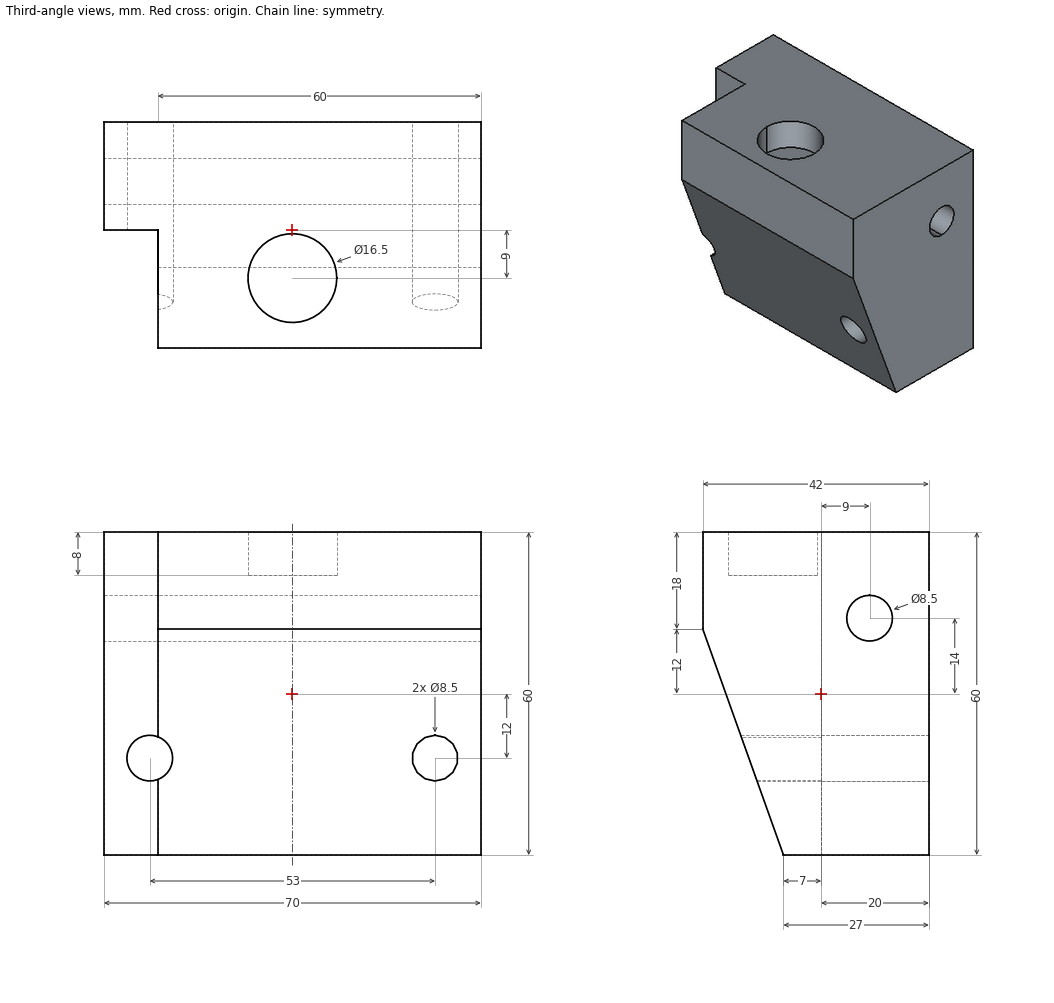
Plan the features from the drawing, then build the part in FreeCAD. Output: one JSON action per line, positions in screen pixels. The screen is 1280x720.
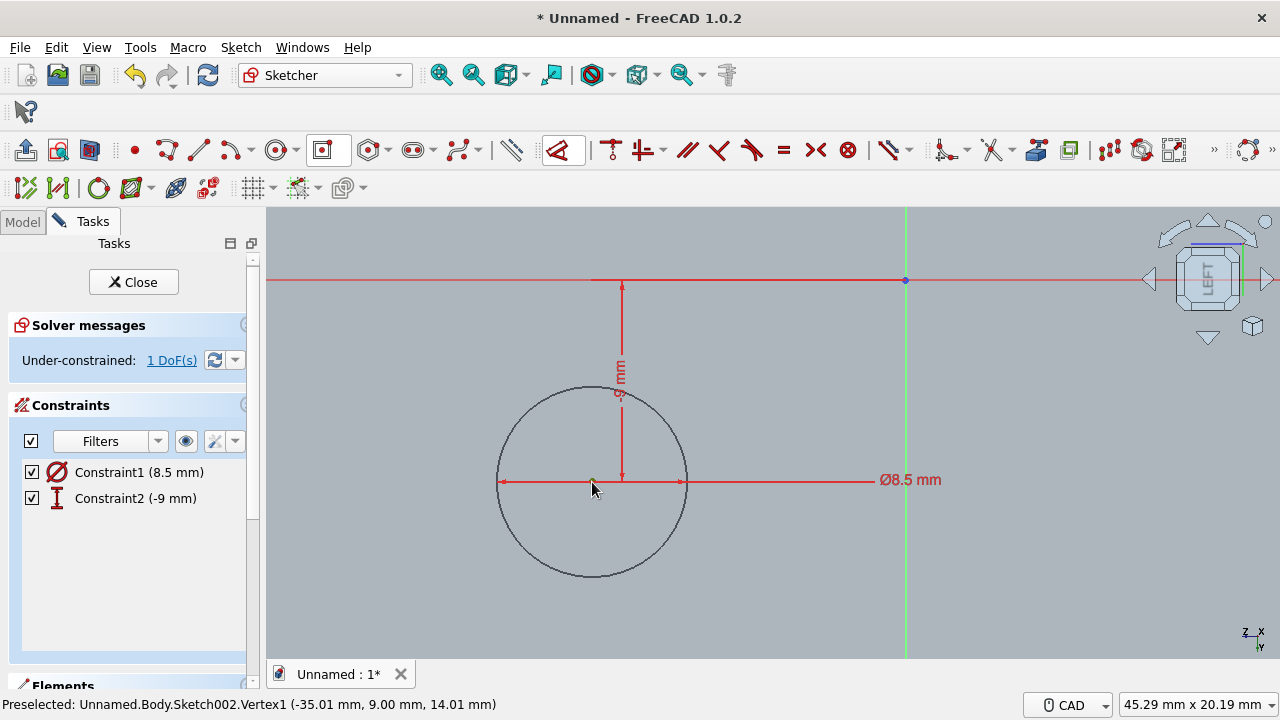
{"action": "key", "text": "l"}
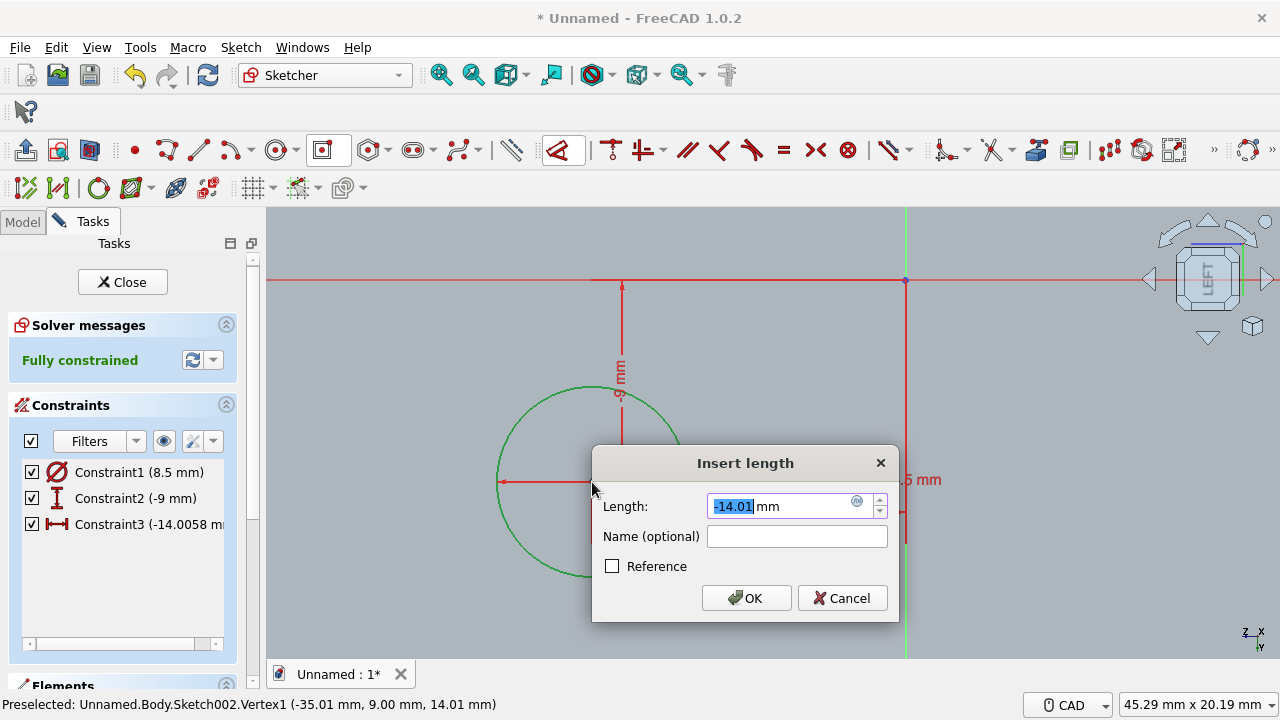
{"action": "type", "text": "-14"}
{"action": "key", "text": "Return"}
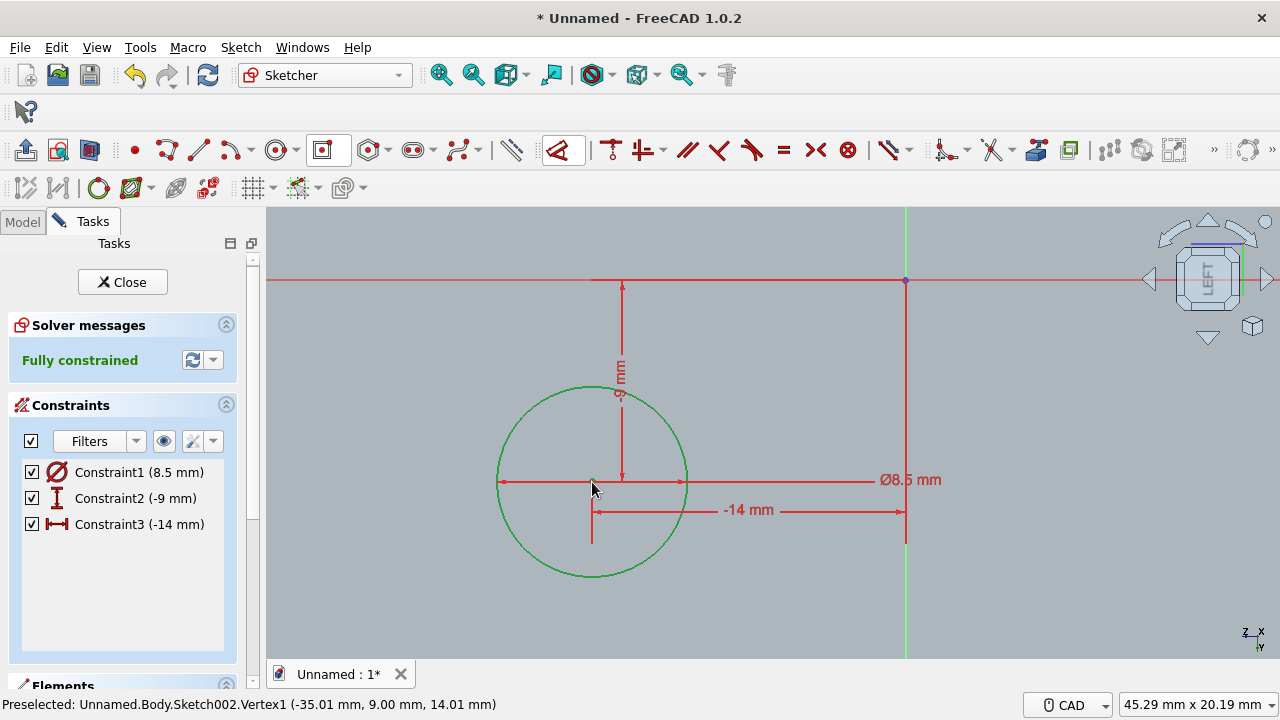
{"action": "left_click", "coordinate": [123, 282]}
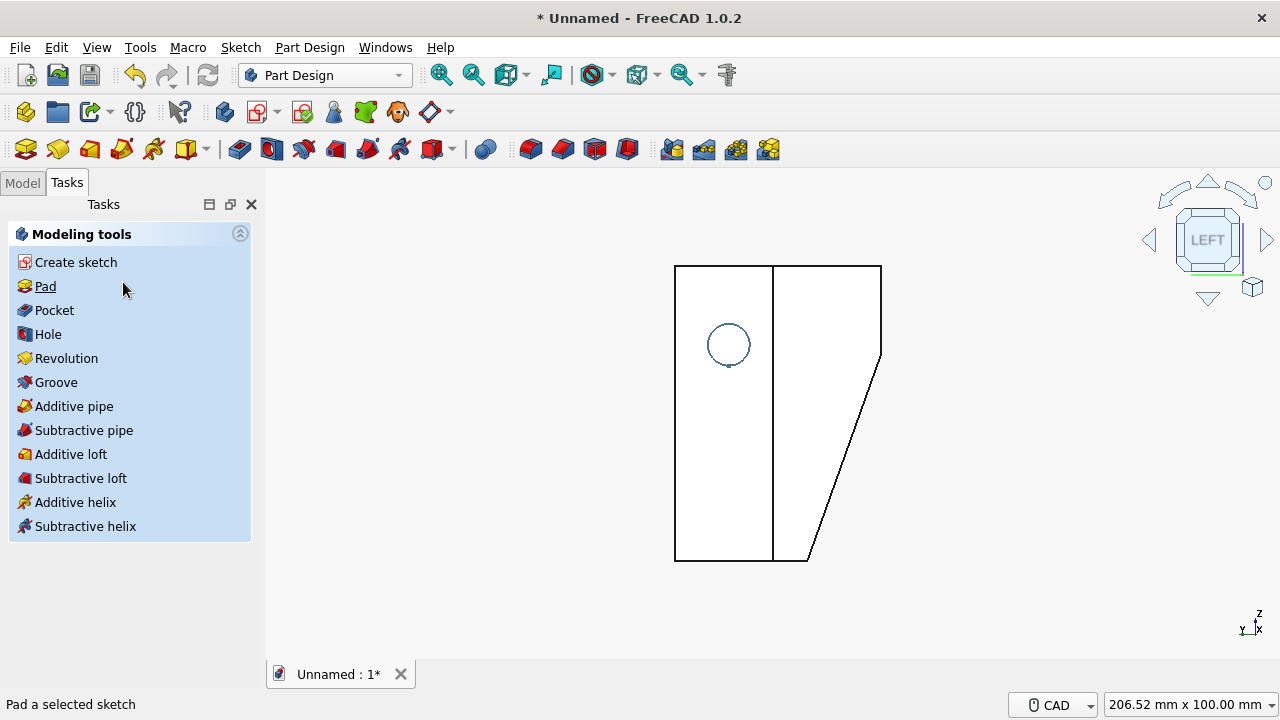
{"action": "left_click", "coordinate": [240, 150]}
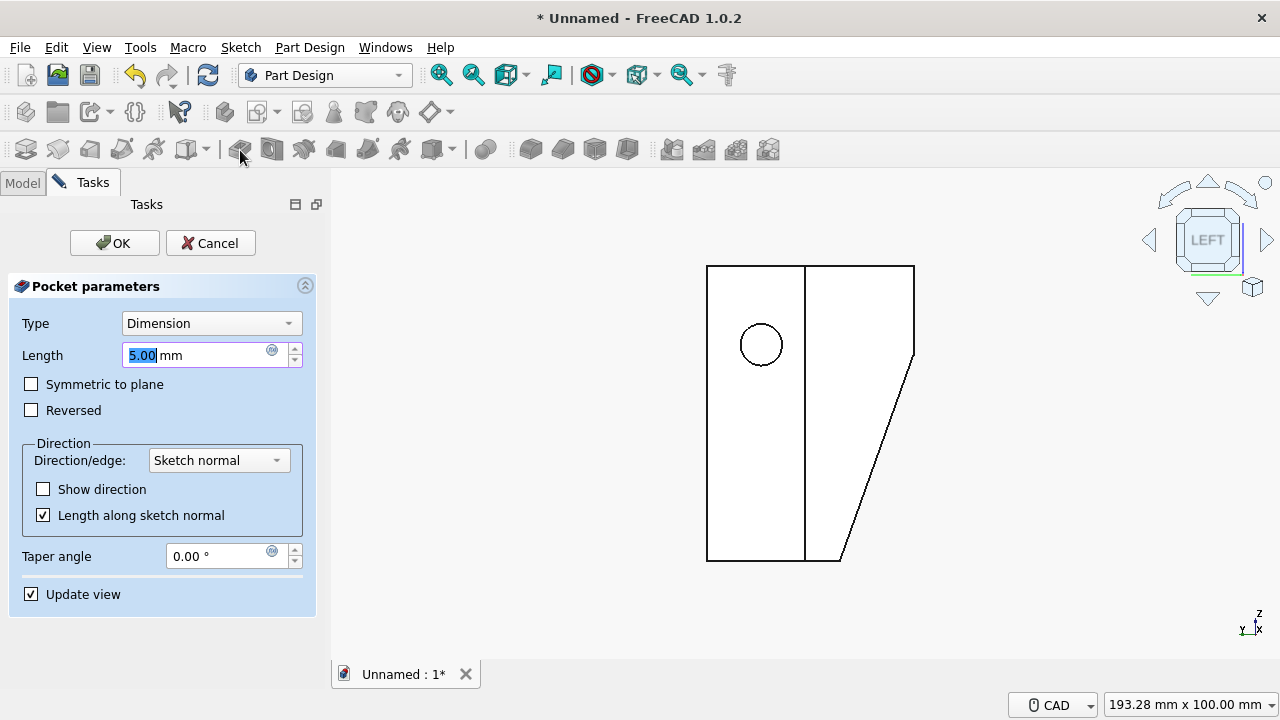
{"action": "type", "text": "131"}
{"action": "key", "text": "Tab"}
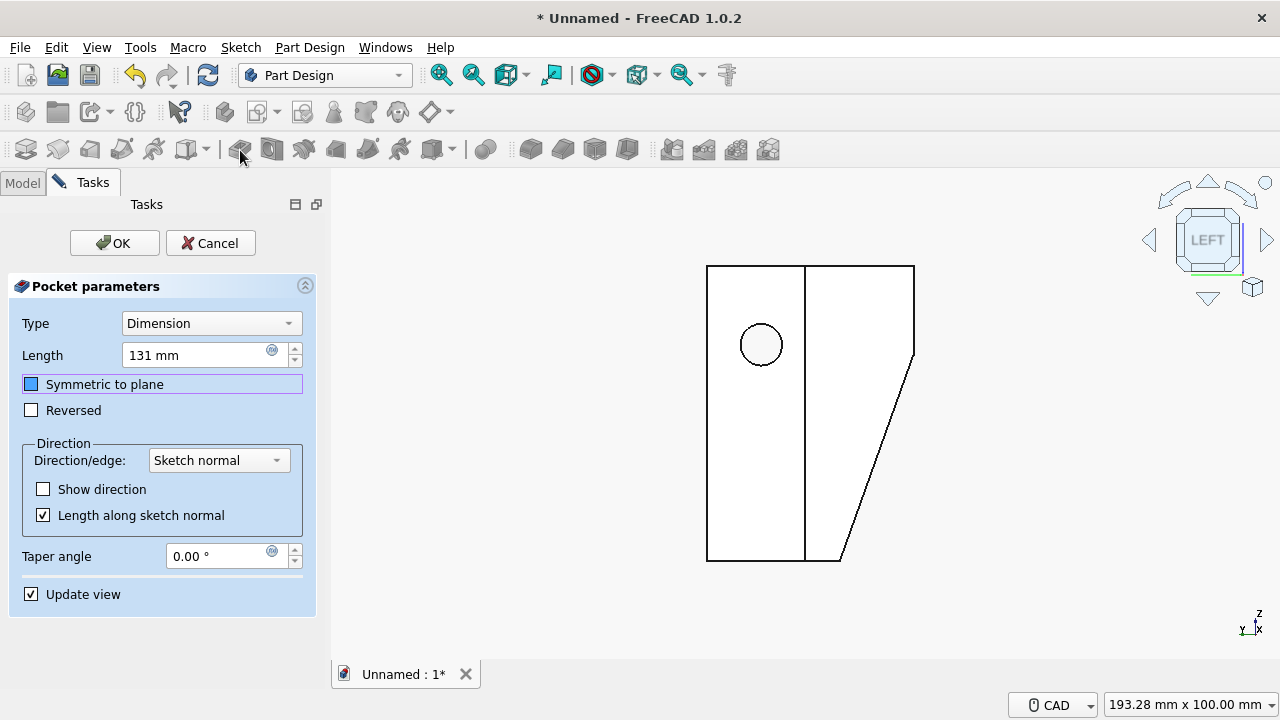
{"action": "left_click", "coordinate": [115, 243]}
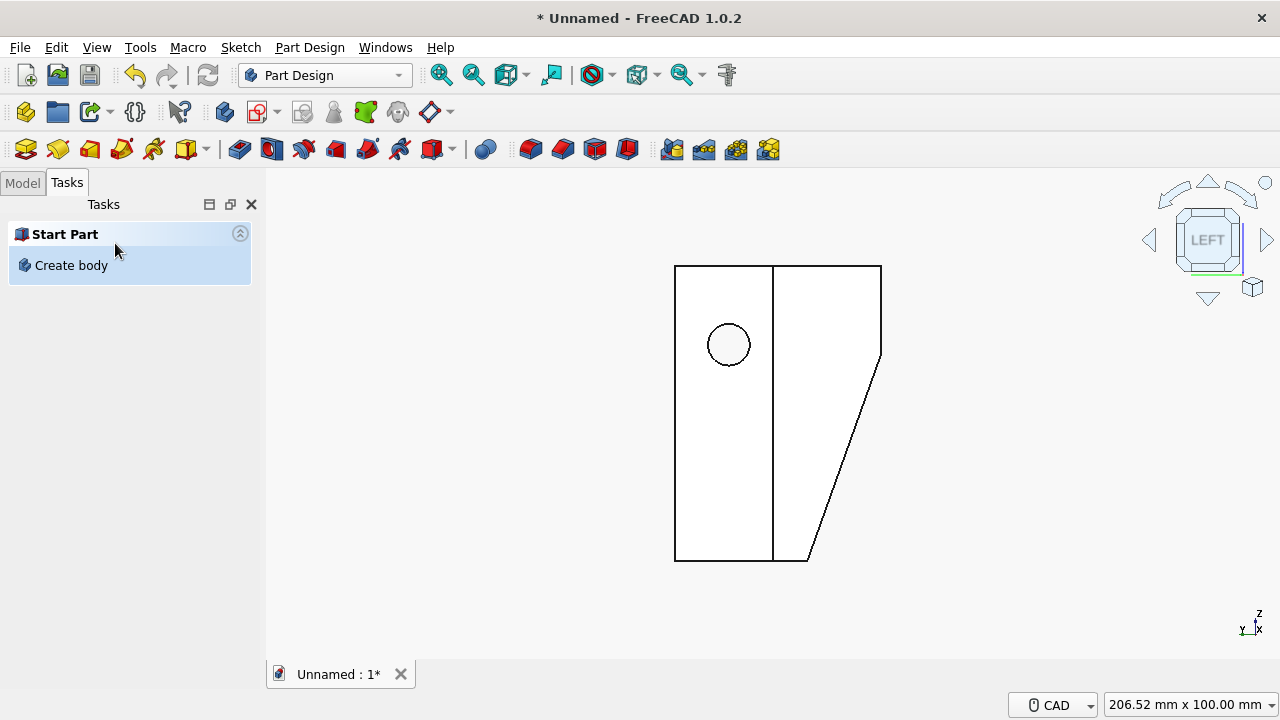
{"action": "key", "text": "4"}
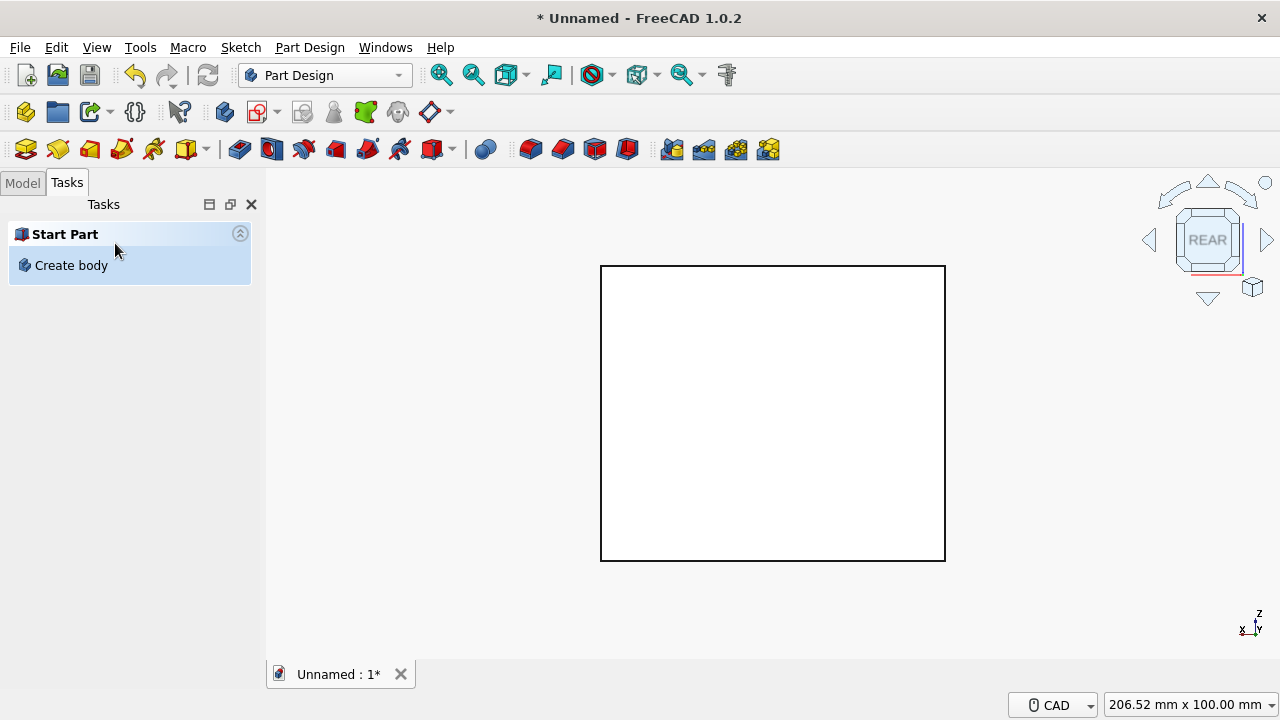
{"action": "left_click", "coordinate": [773, 413]}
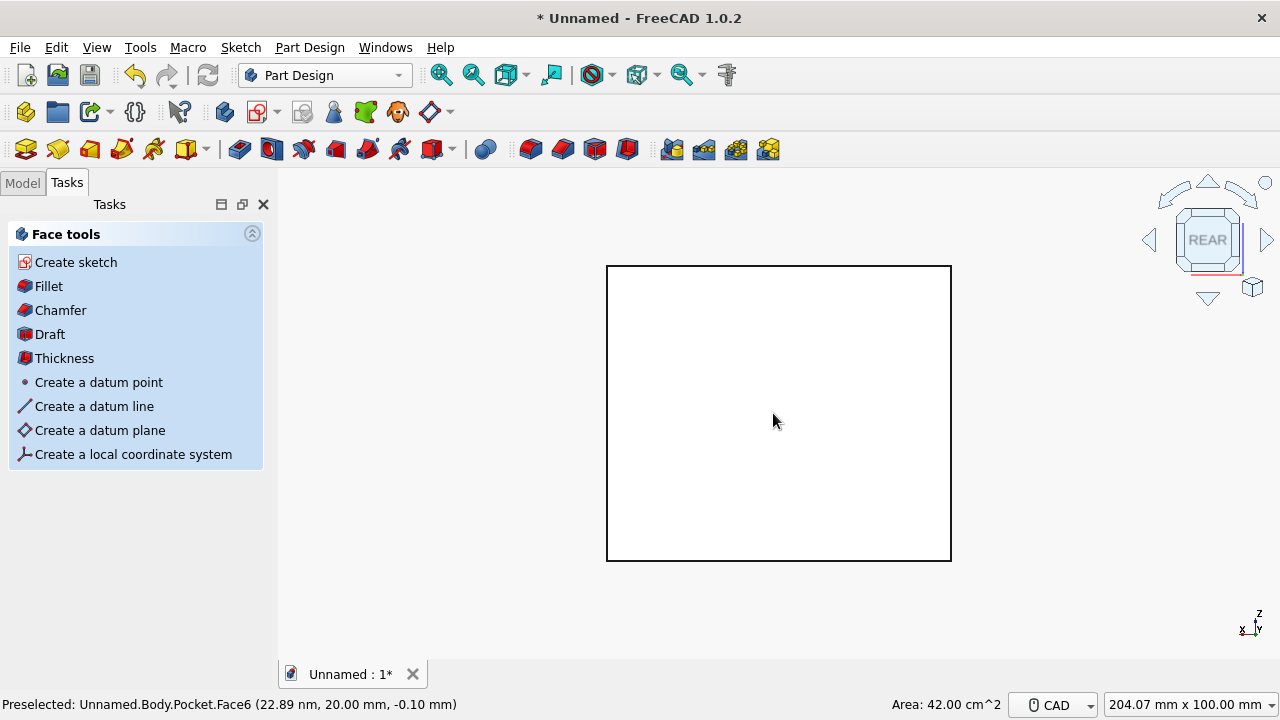
{"action": "left_click", "coordinate": [258, 112]}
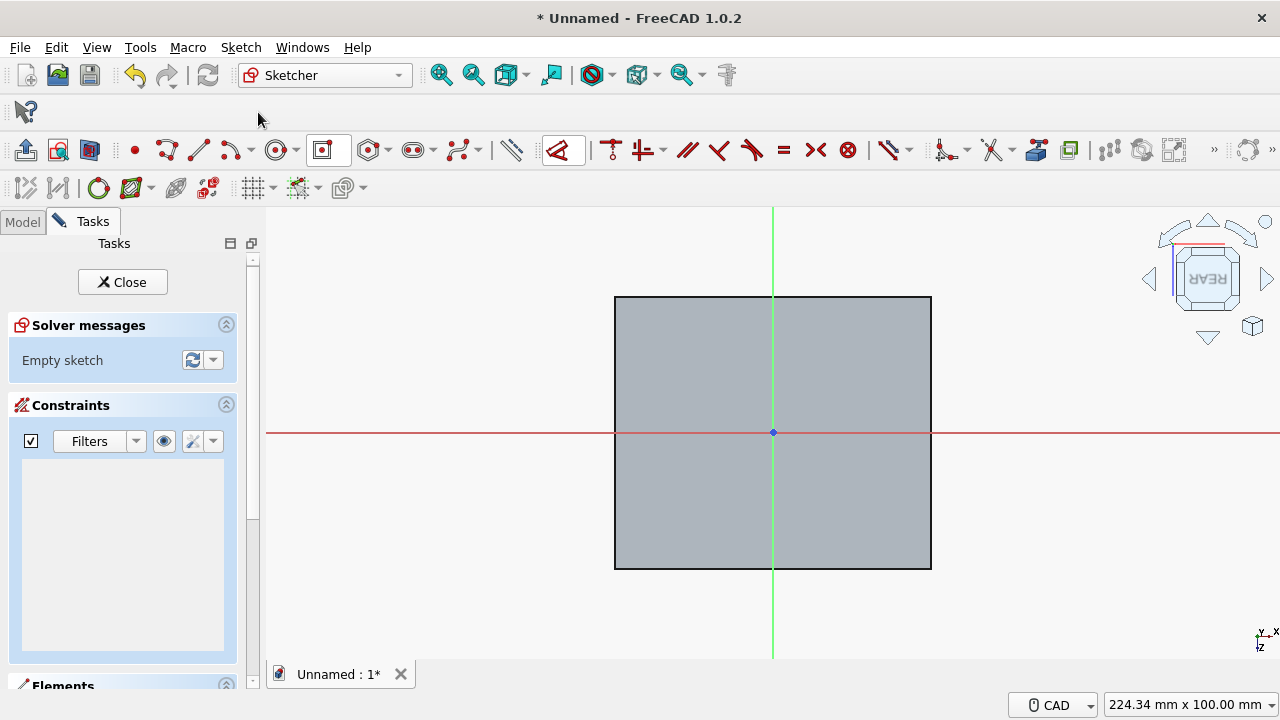
{"action": "scroll", "coordinate": [829, 366], "scroll_direction": "up", "scroll_amount": 4}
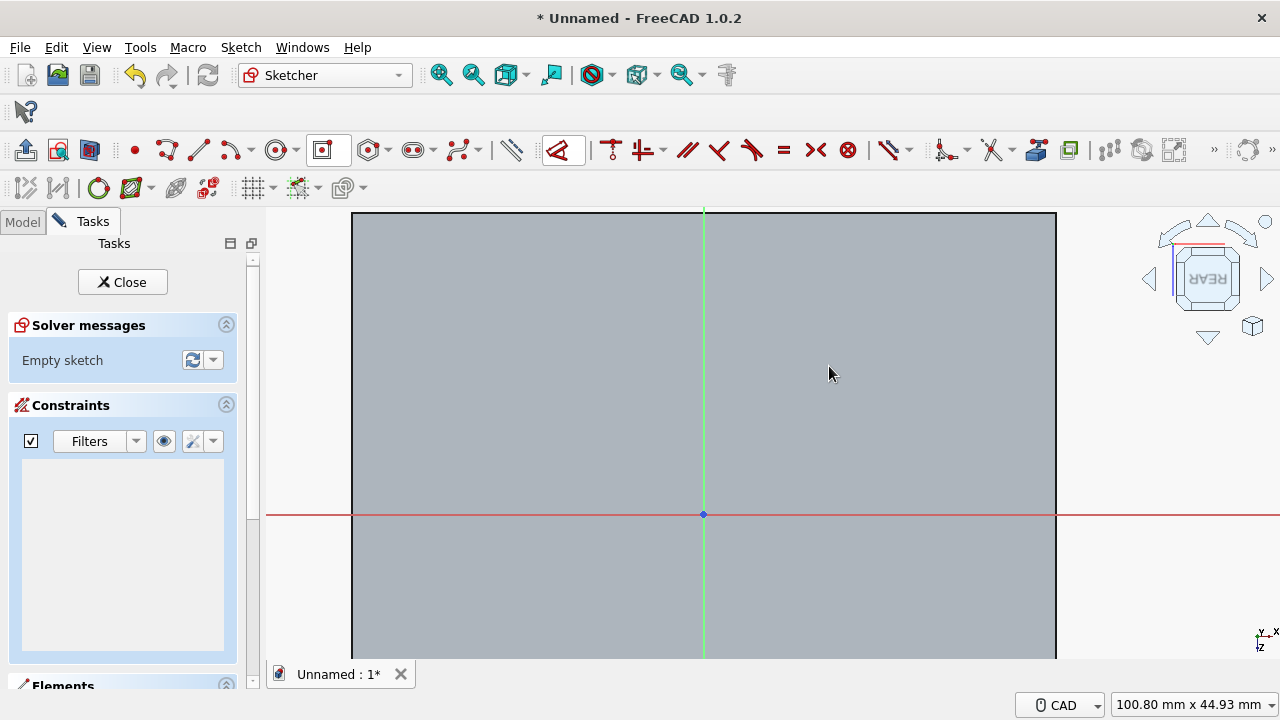
{"action": "left_click", "coordinate": [276, 150]}